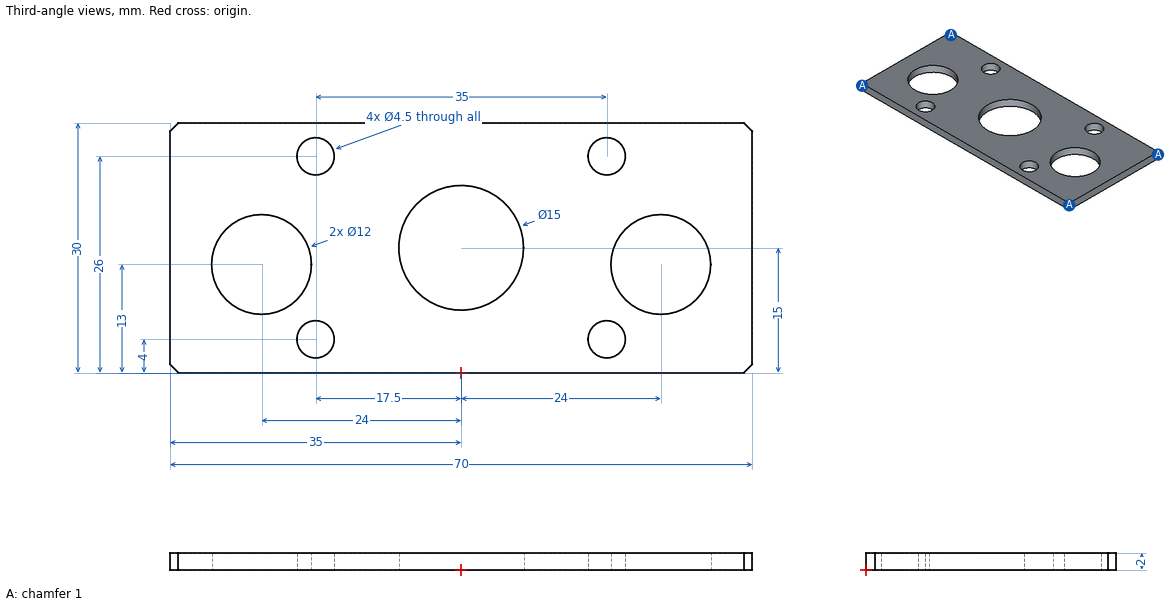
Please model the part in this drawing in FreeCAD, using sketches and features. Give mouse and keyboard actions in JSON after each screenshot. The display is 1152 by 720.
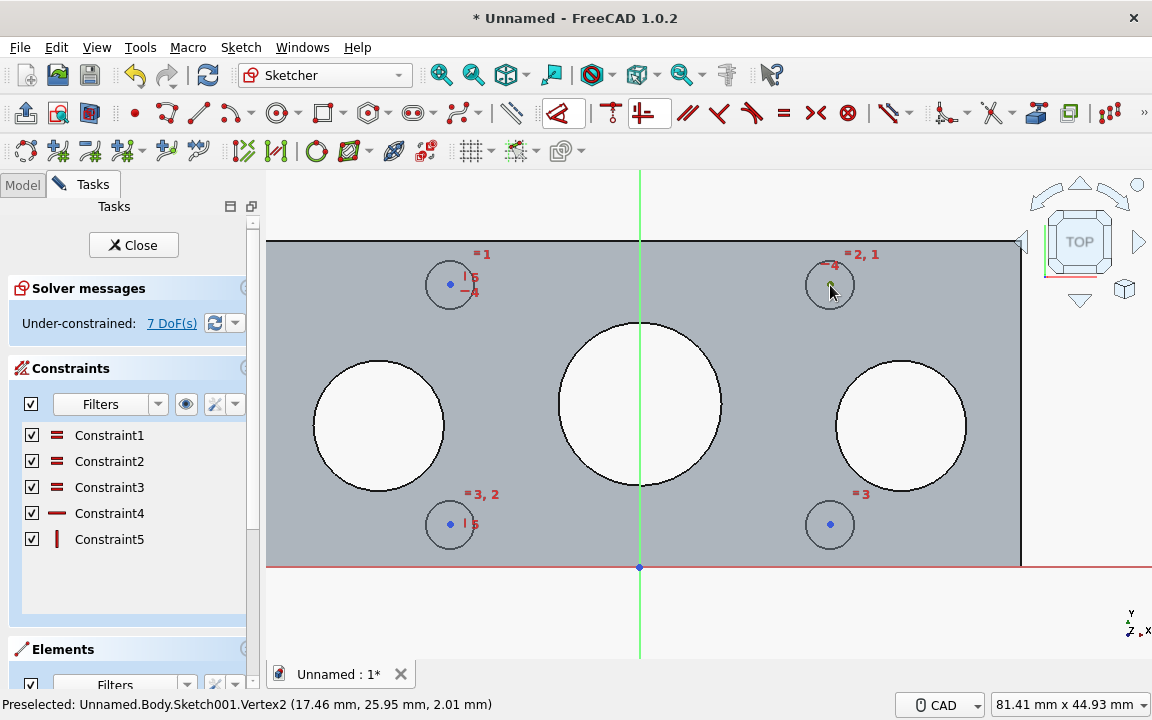
{"action": "left_click", "coordinate": [830, 525]}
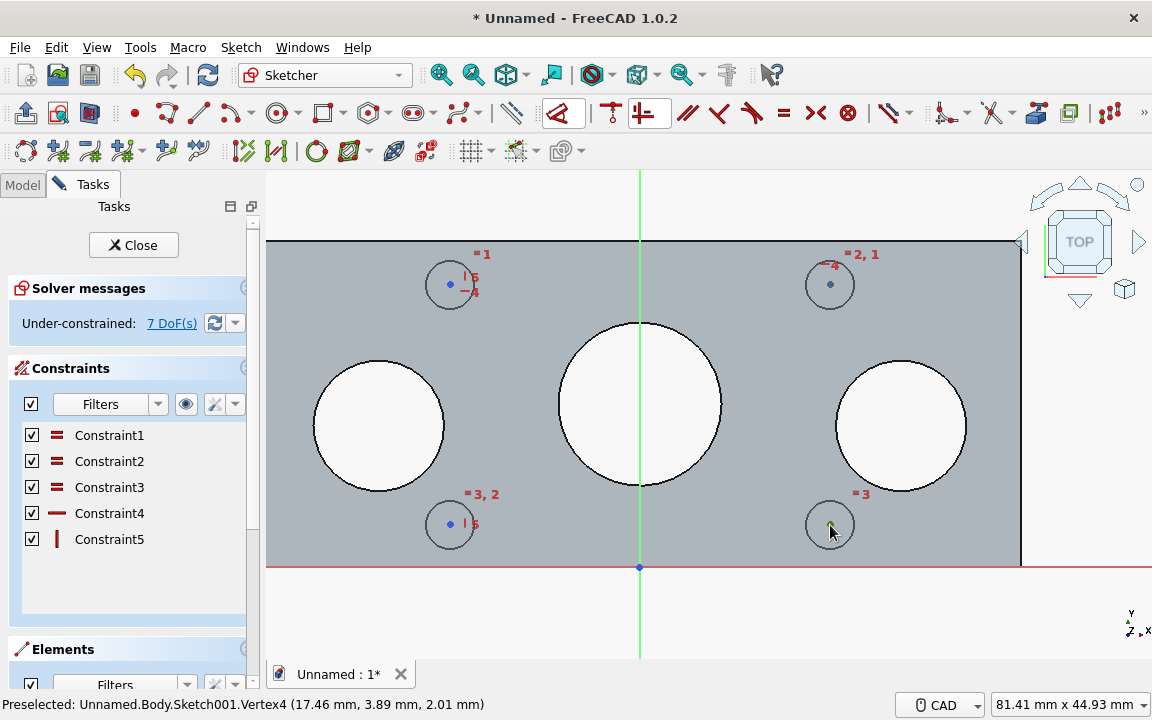
{"action": "left_click", "coordinate": [666, 114]}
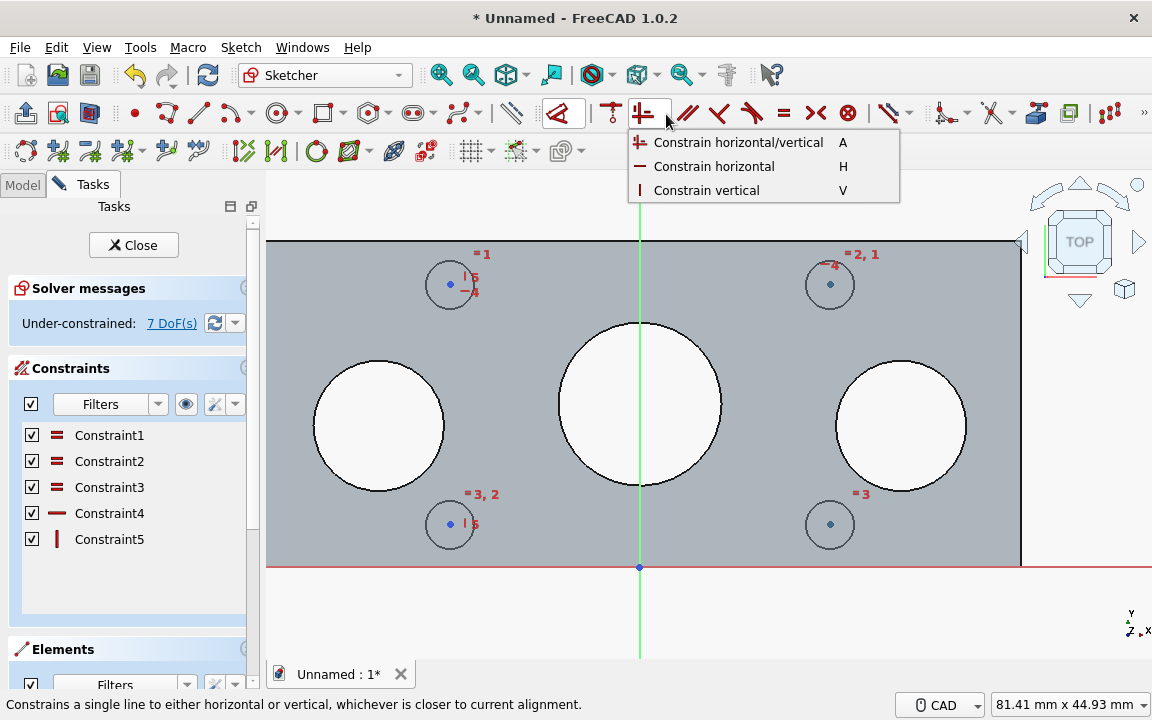
{"action": "left_click", "coordinate": [764, 190]}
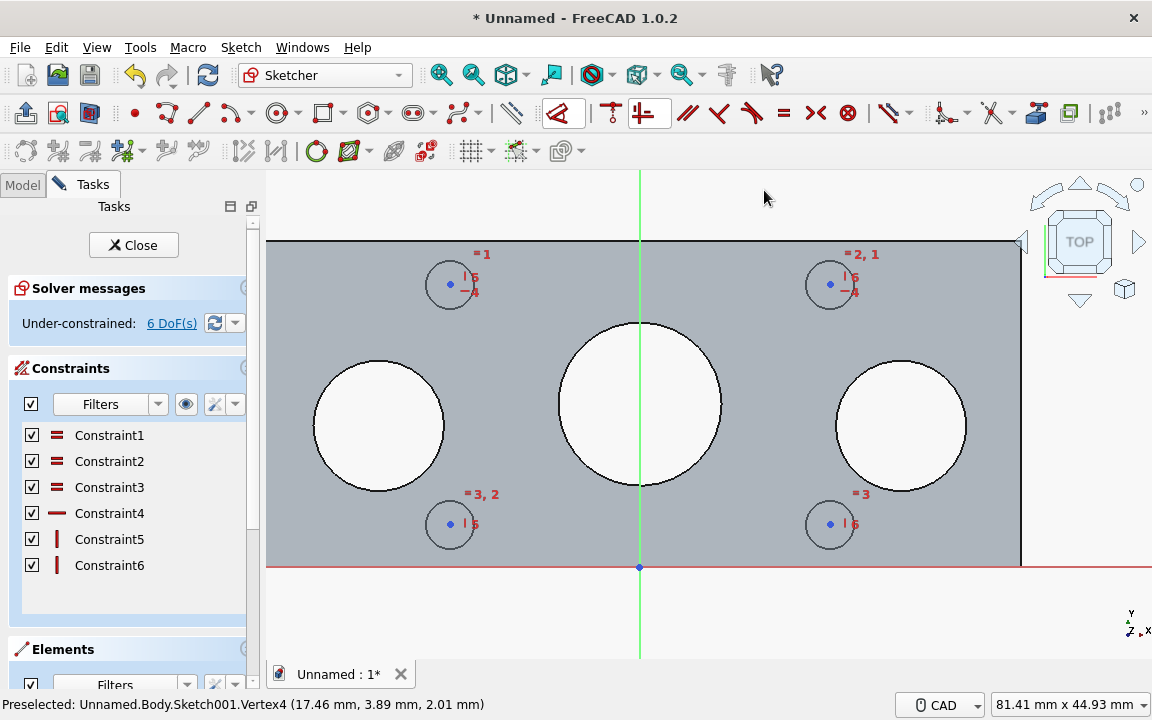
{"action": "left_click", "coordinate": [450, 525]}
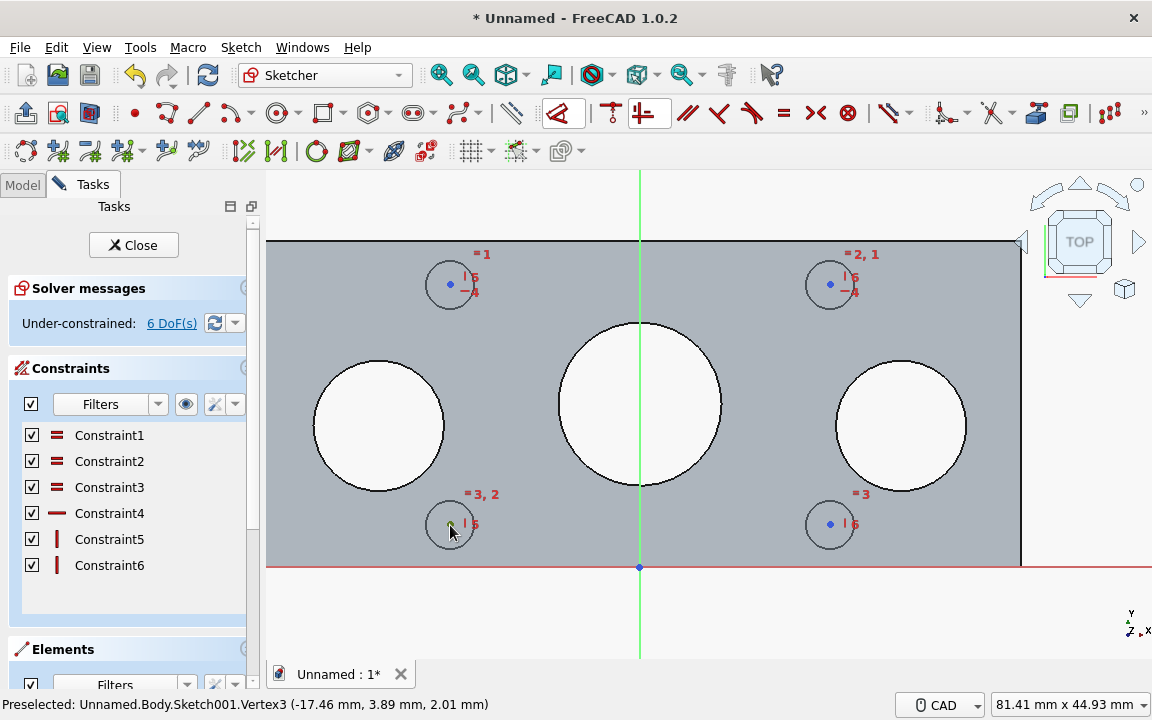
{"action": "left_click", "coordinate": [830, 525]}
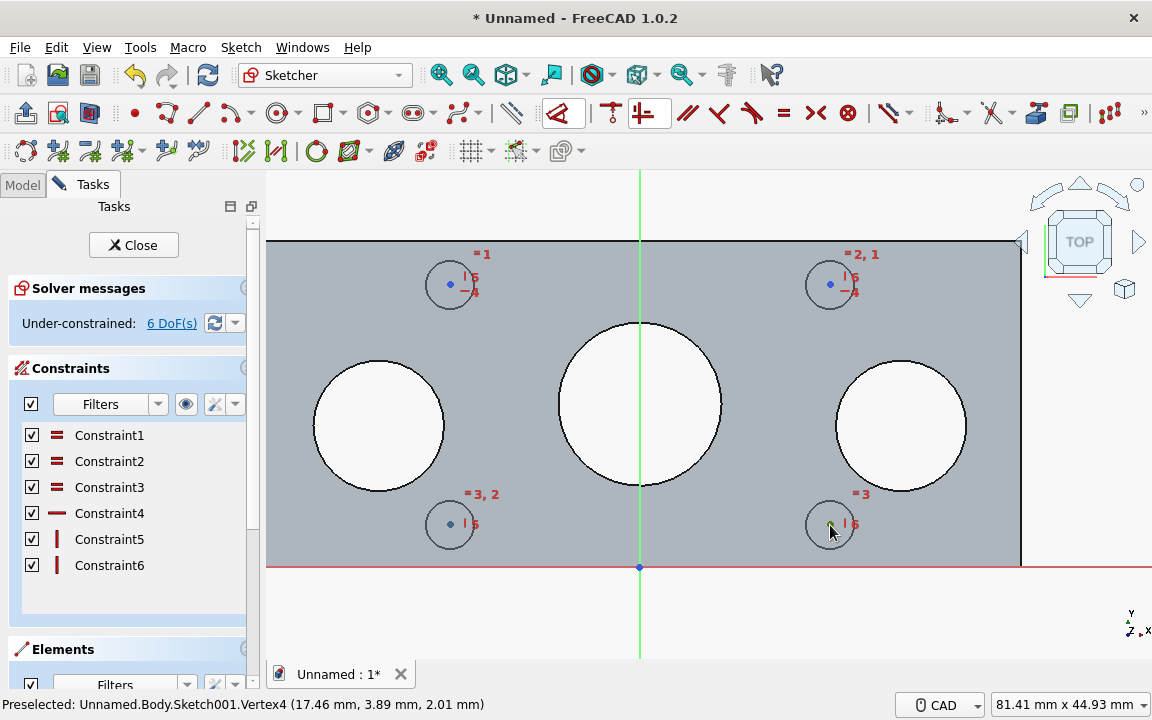
{"action": "key", "text": "h"}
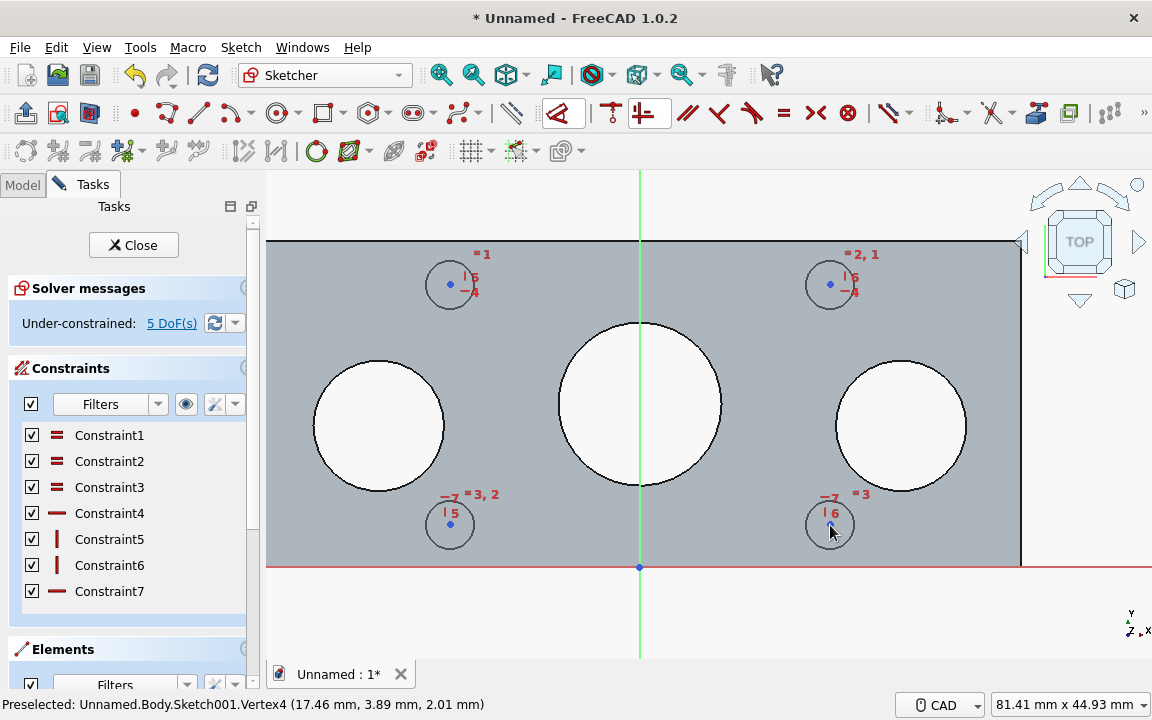
{"action": "left_click", "coordinate": [467, 268]}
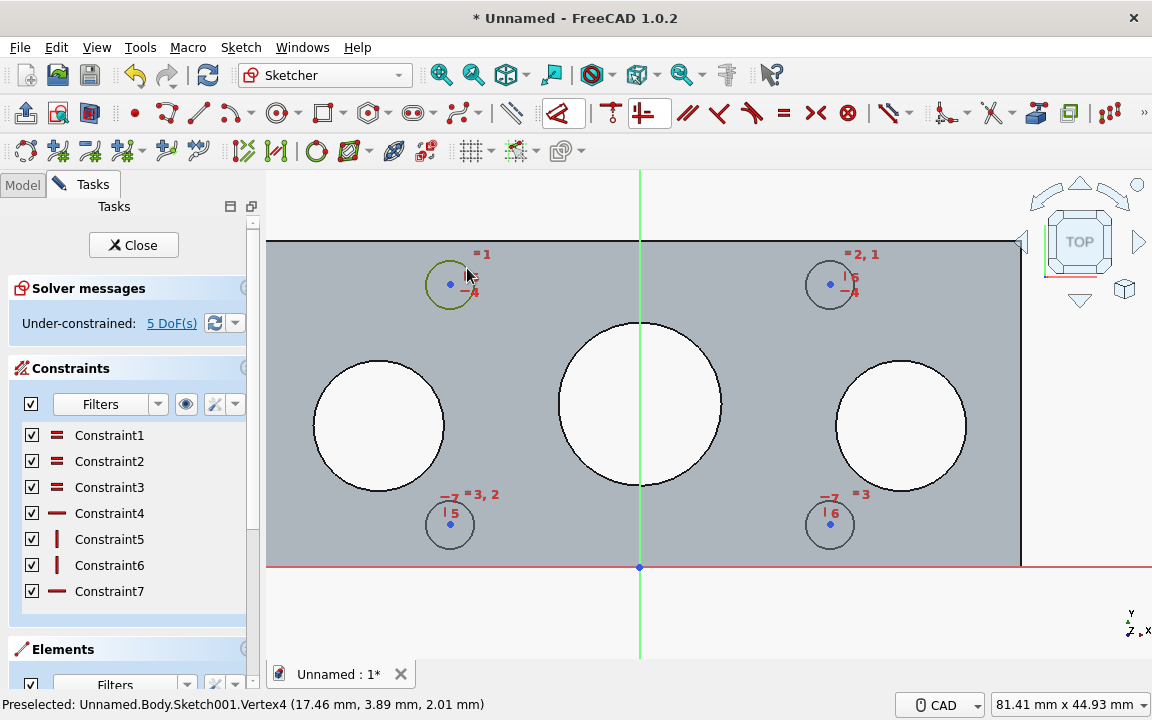
{"action": "left_click", "coordinate": [580, 114]}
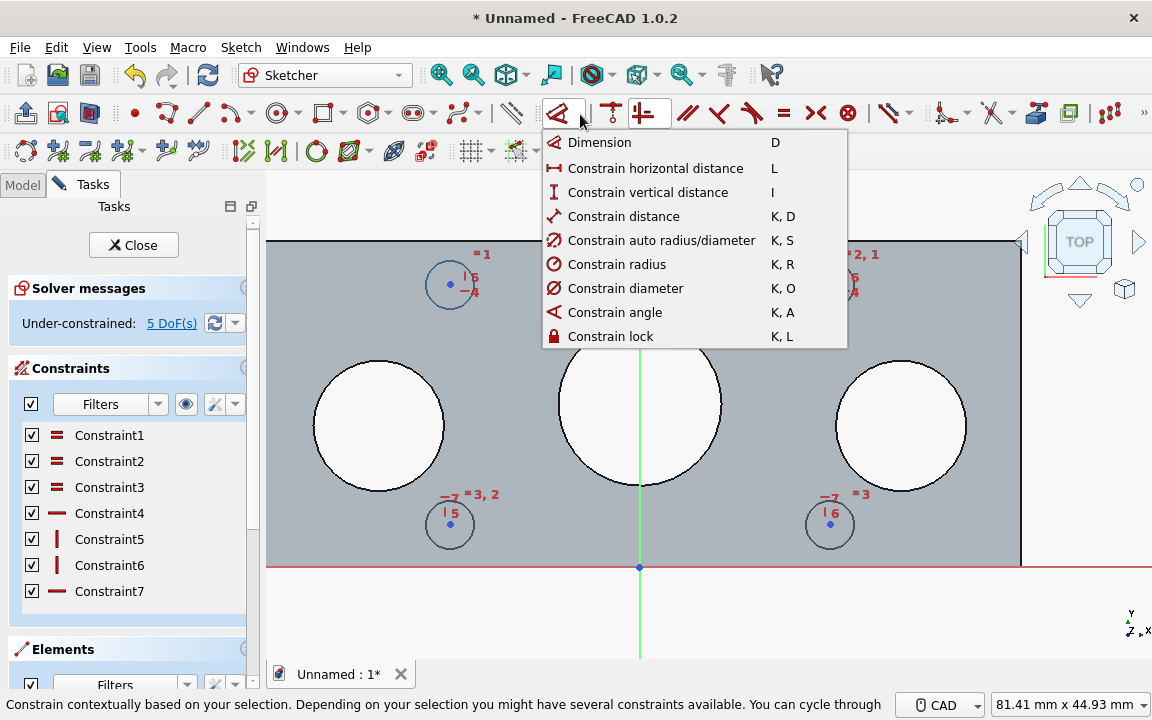
{"action": "left_click", "coordinate": [695, 288]}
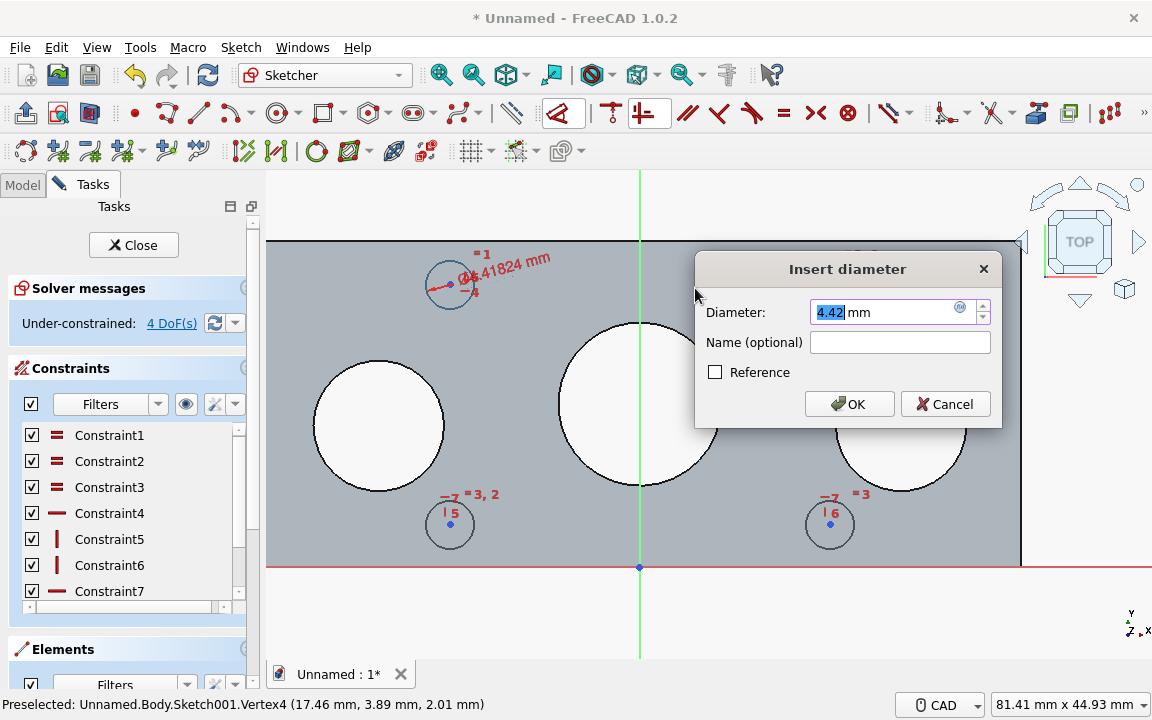
{"action": "type", "text": "4.5"}
{"action": "key", "text": "Return"}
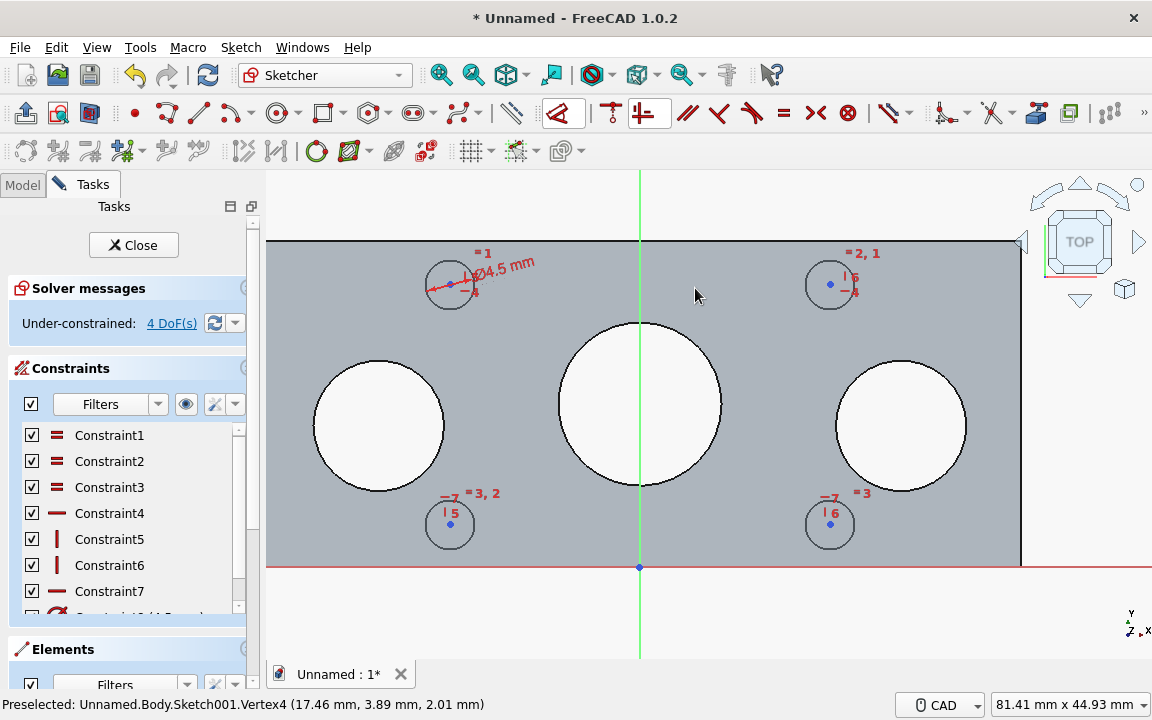
{"action": "left_click", "coordinate": [450, 525]}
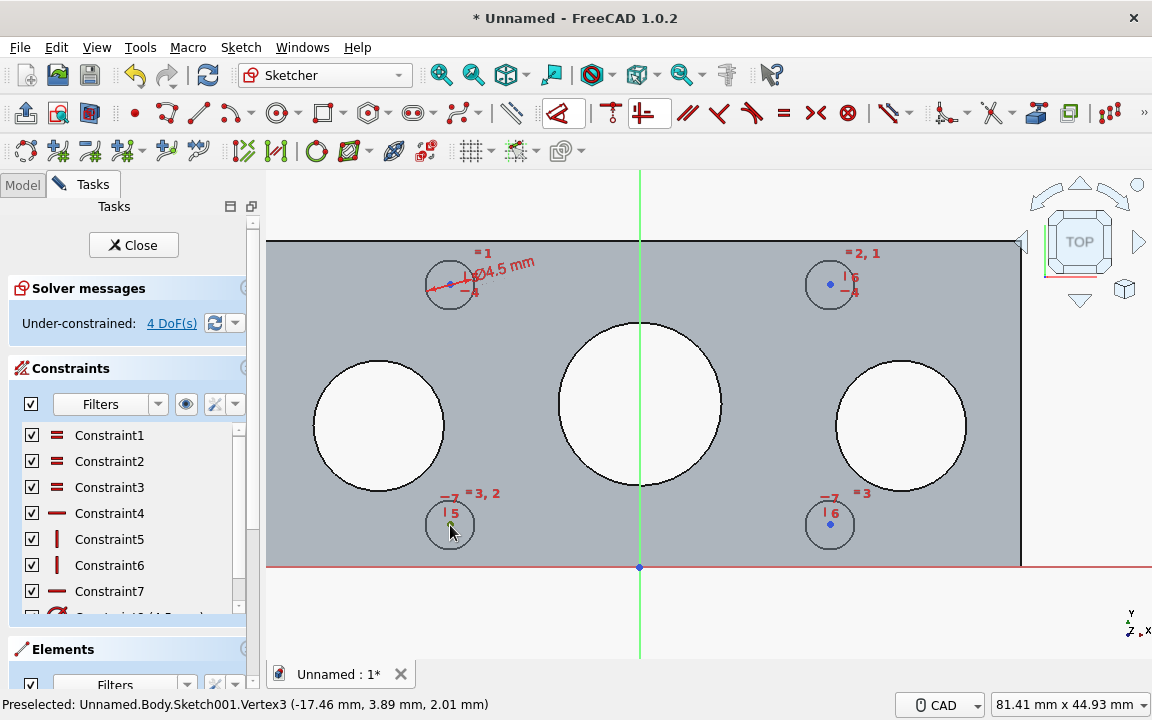
{"action": "key", "text": "i"}